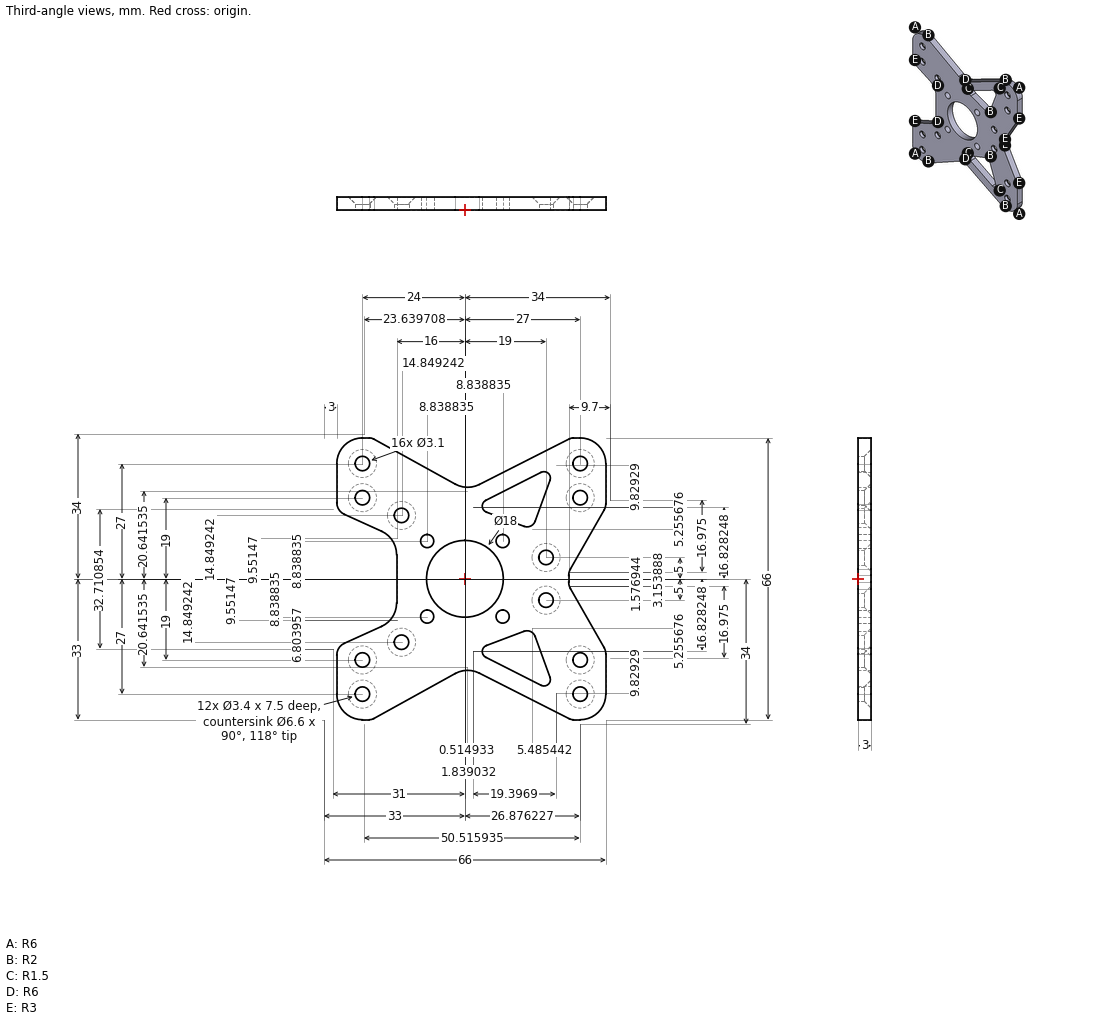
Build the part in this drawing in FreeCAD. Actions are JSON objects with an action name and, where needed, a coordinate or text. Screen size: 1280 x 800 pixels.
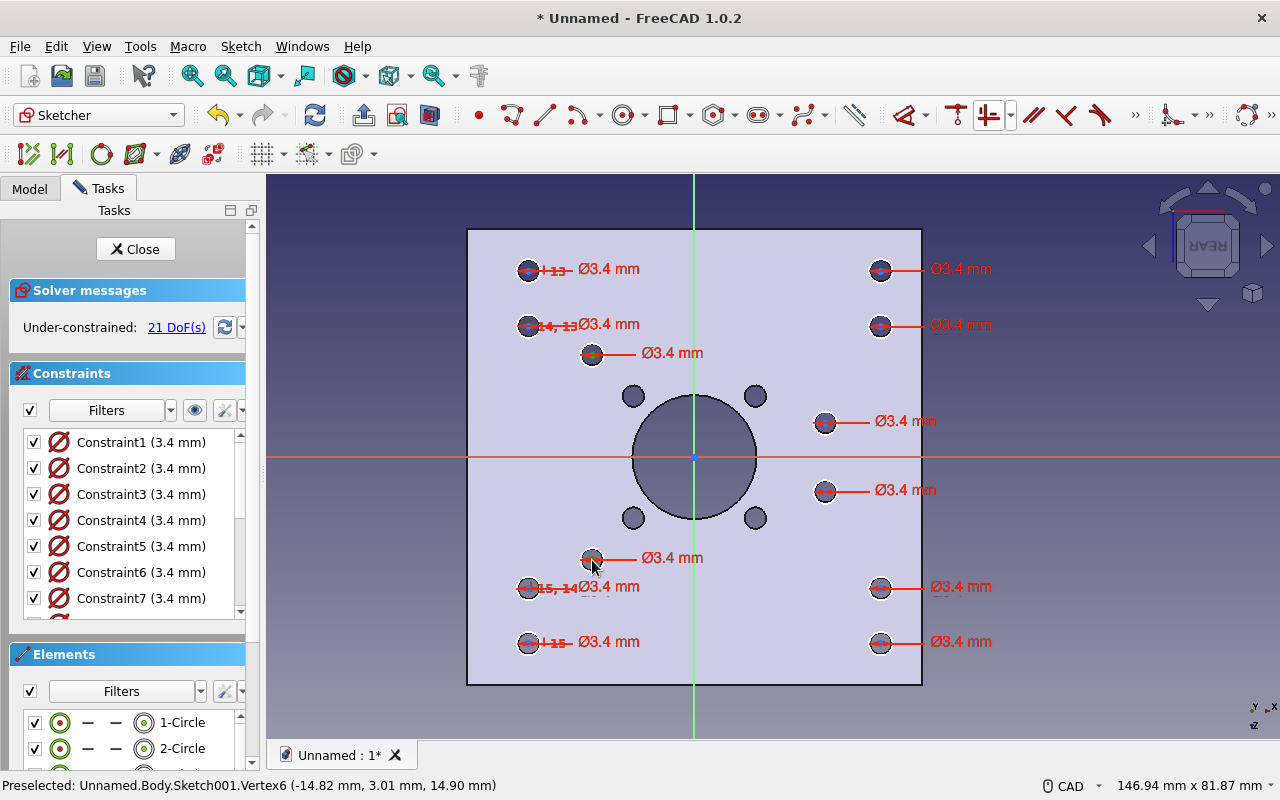
{"action": "key", "text": "v"}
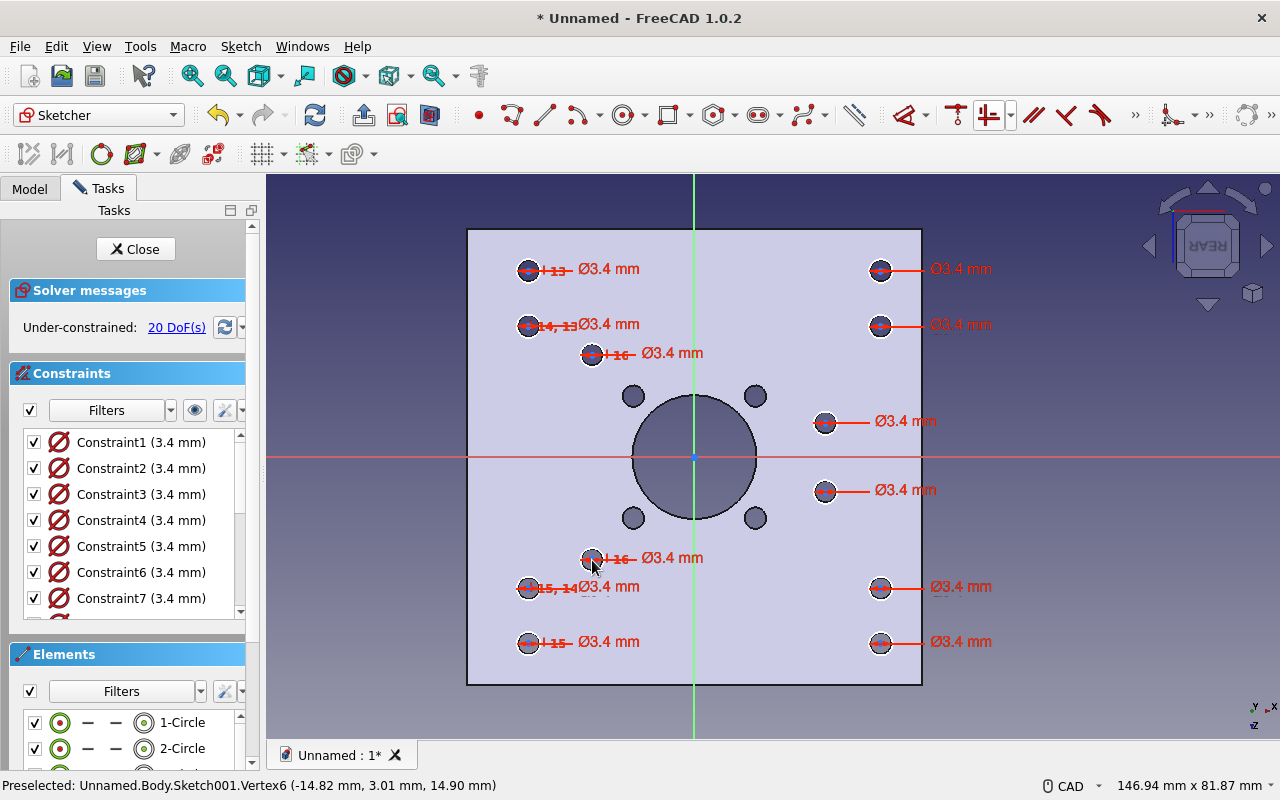
{"action": "left_click", "coordinate": [825, 492]}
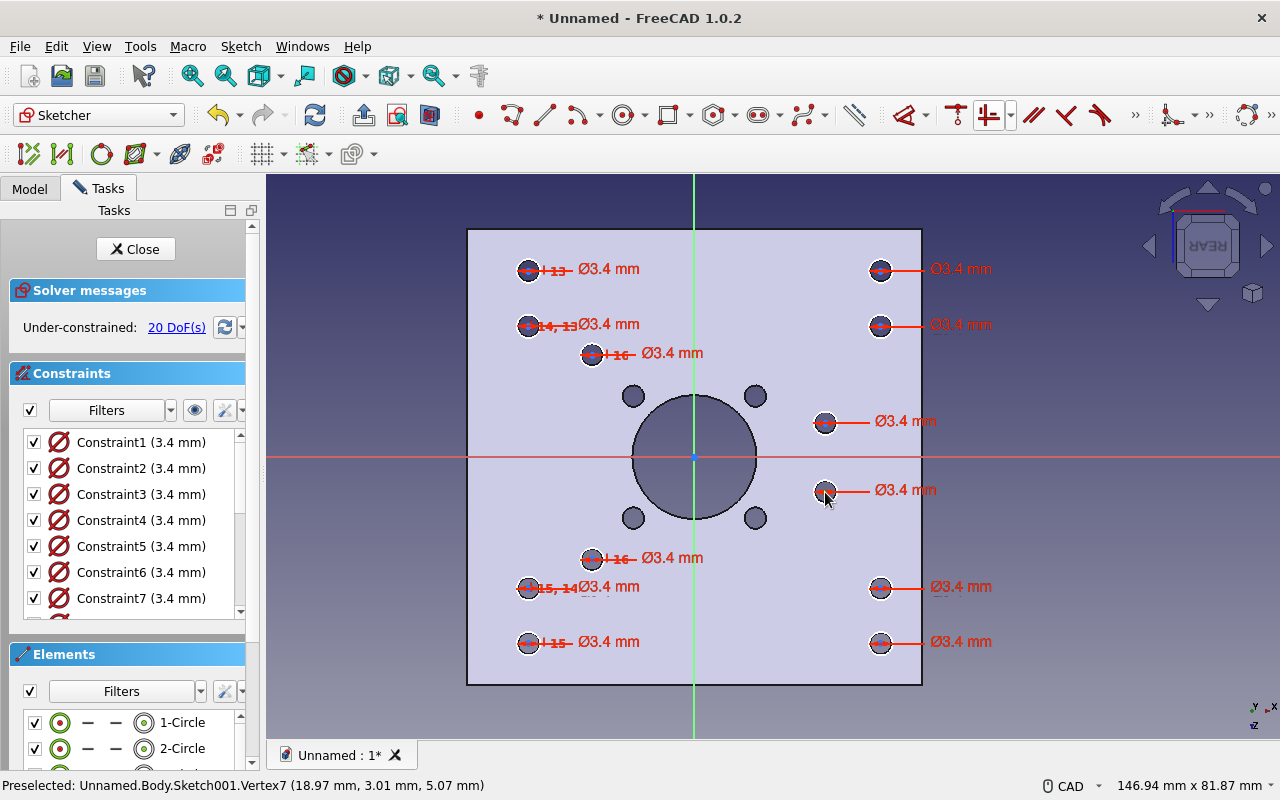
{"action": "left_click", "coordinate": [825, 423]}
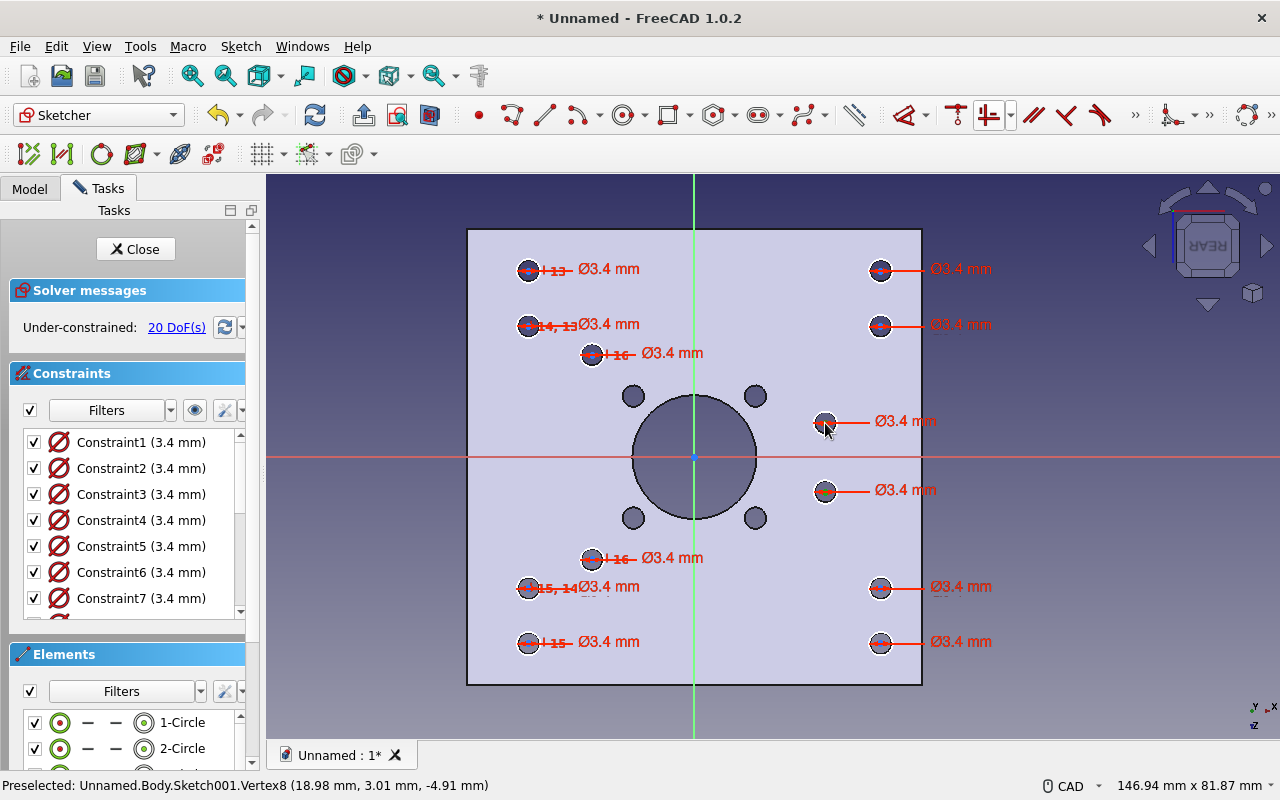
{"action": "key", "text": "v"}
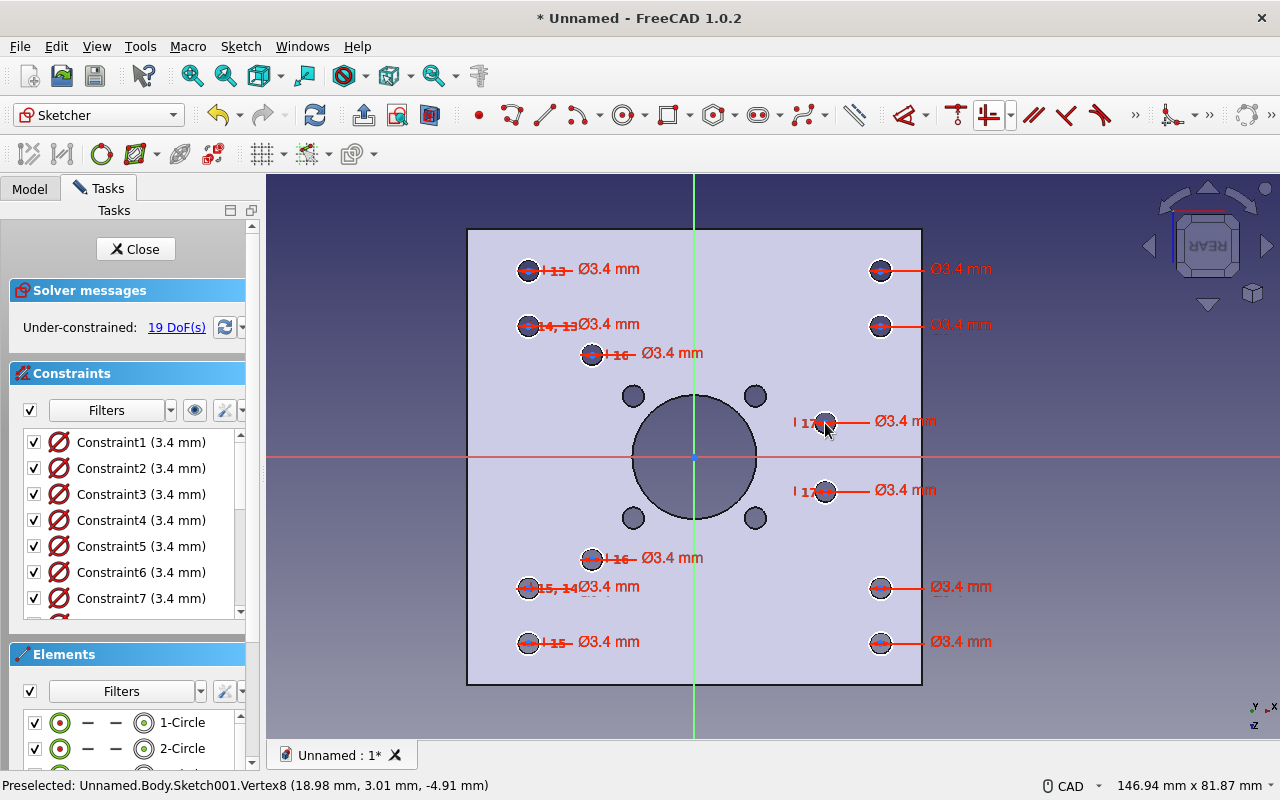
{"action": "left_click", "coordinate": [529, 326]}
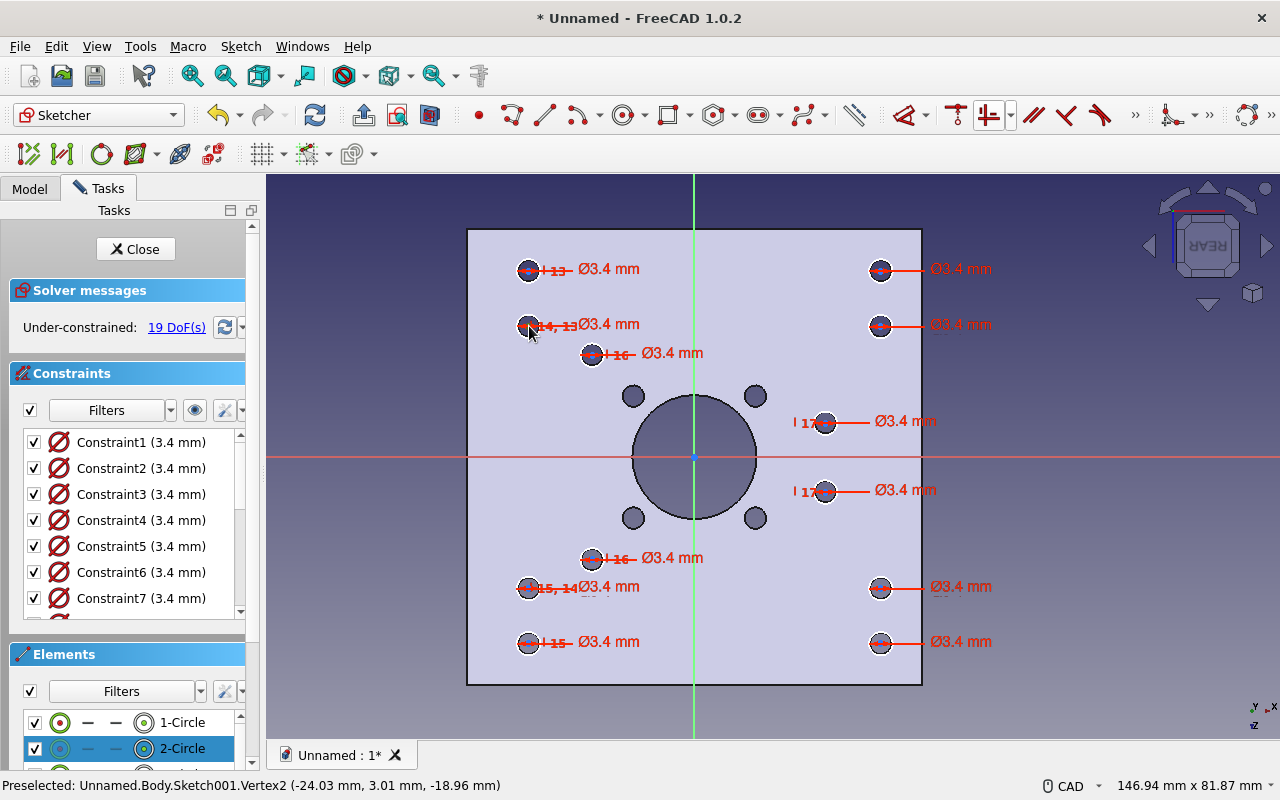
{"action": "left_click", "coordinate": [881, 327]}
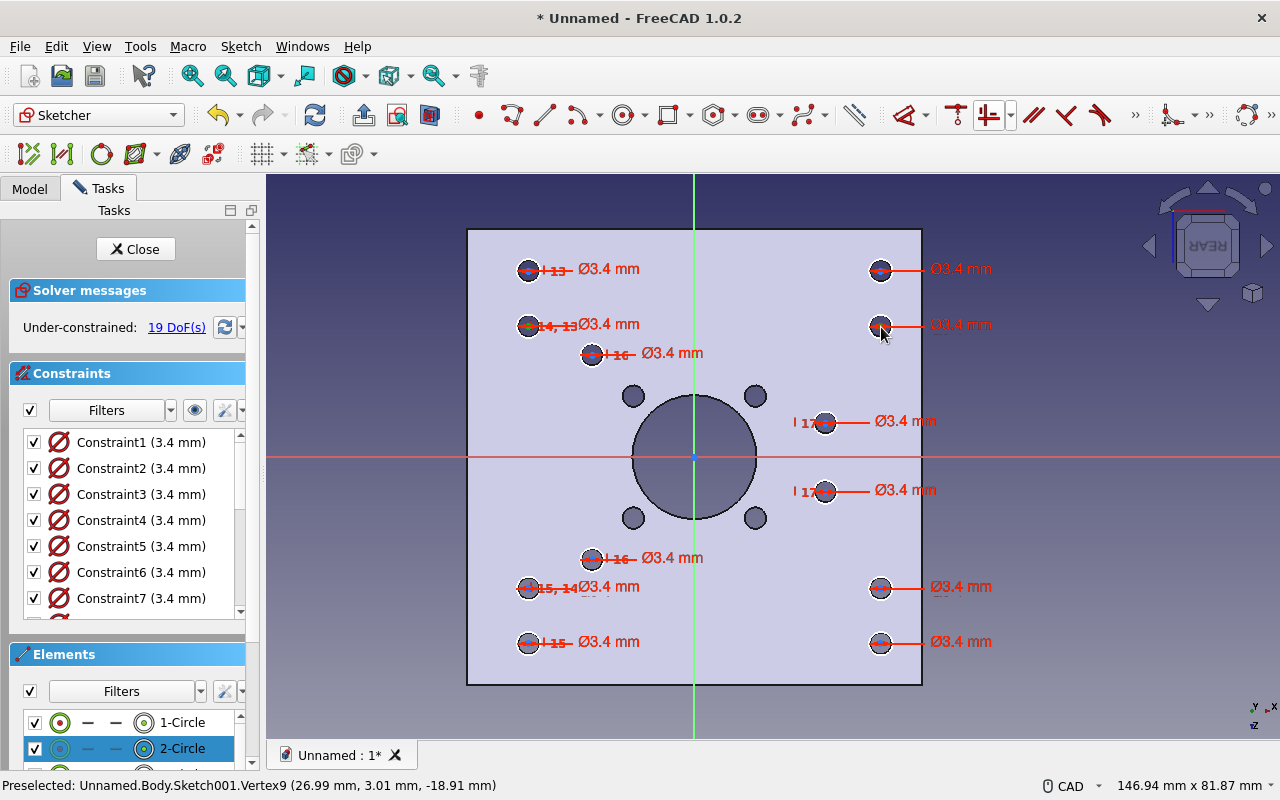
{"action": "left_click", "coordinate": [1010, 116]}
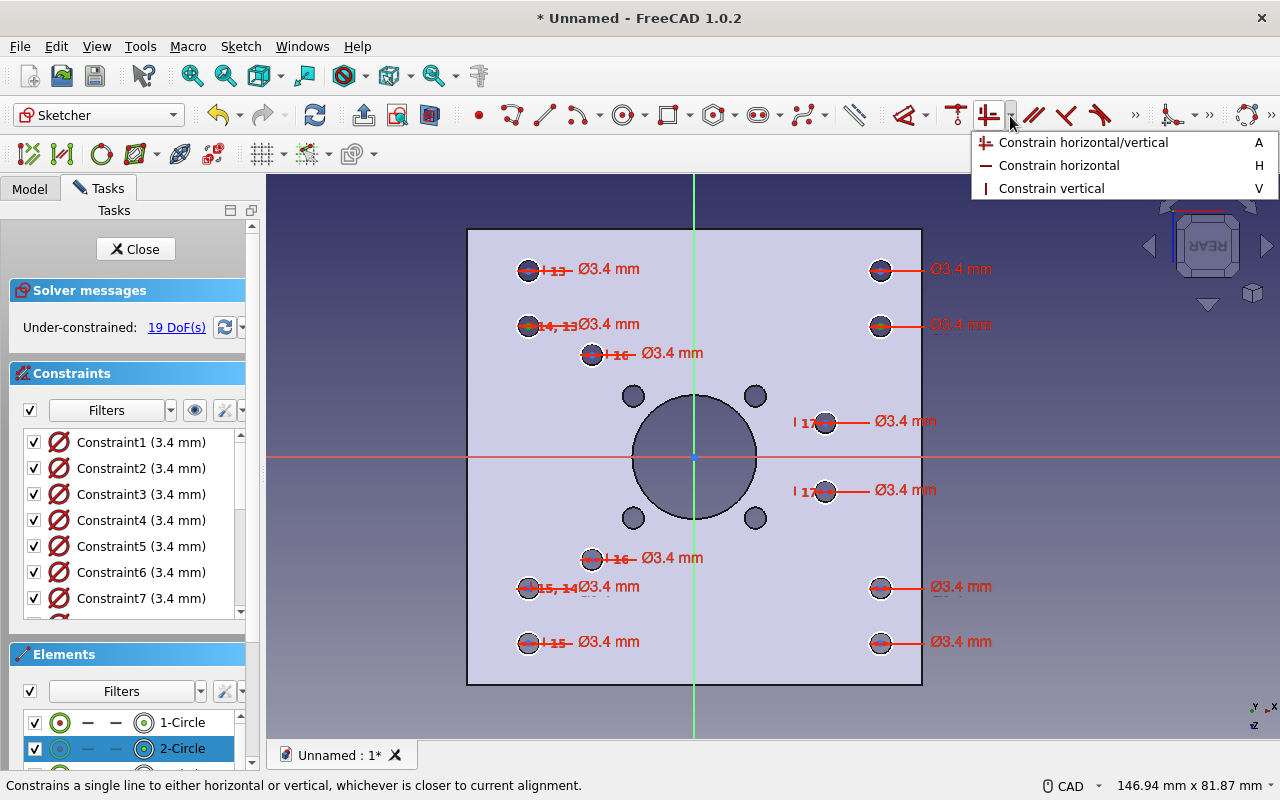
{"action": "left_click", "coordinate": [1125, 166]}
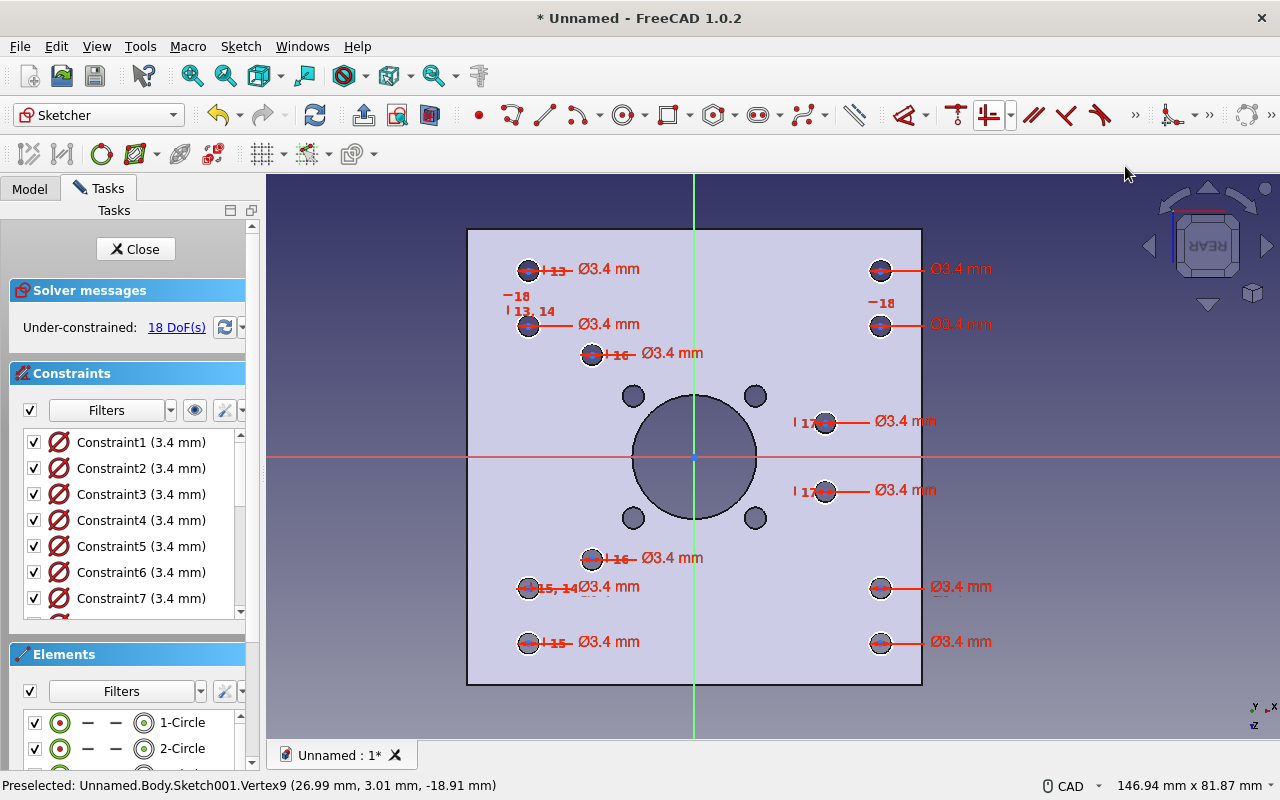
{"action": "left_click", "coordinate": [881, 326]}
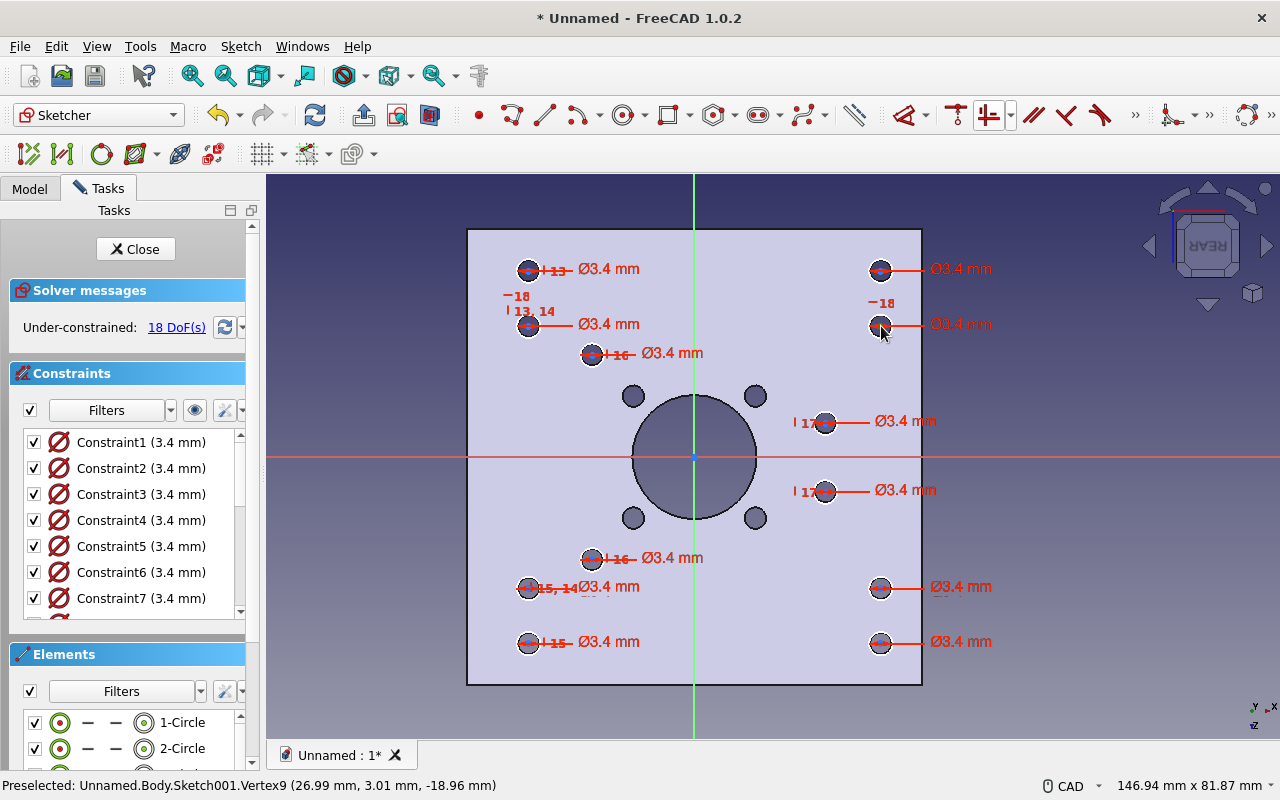
{"action": "left_click", "coordinate": [881, 271]}